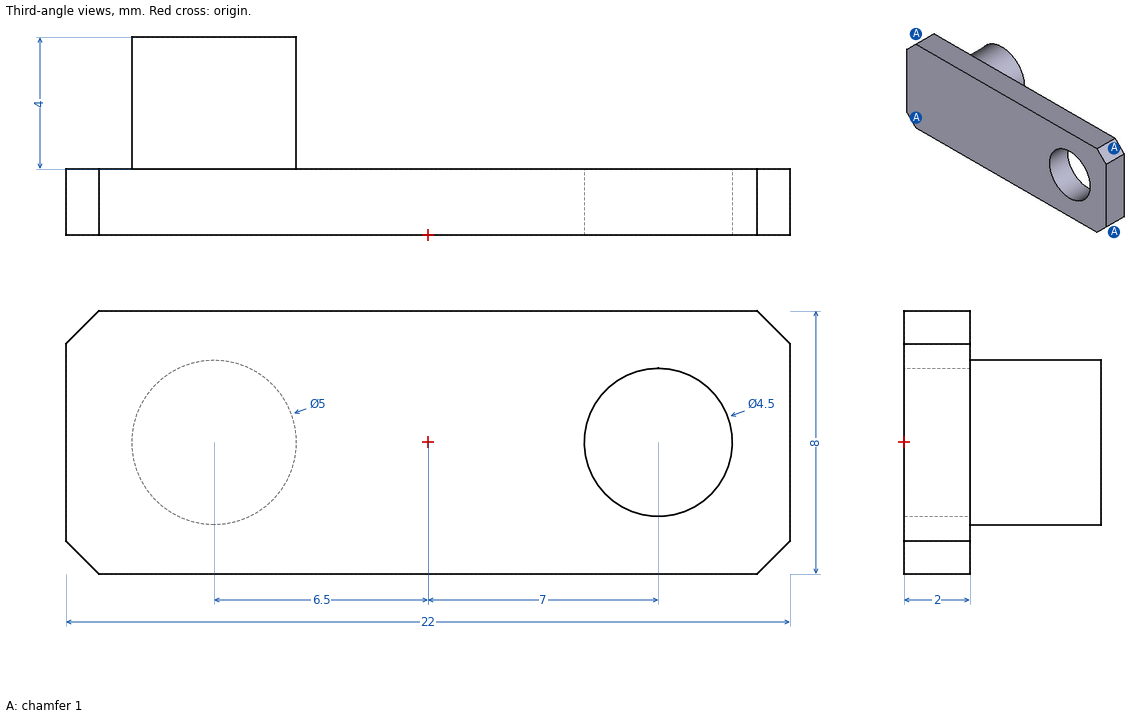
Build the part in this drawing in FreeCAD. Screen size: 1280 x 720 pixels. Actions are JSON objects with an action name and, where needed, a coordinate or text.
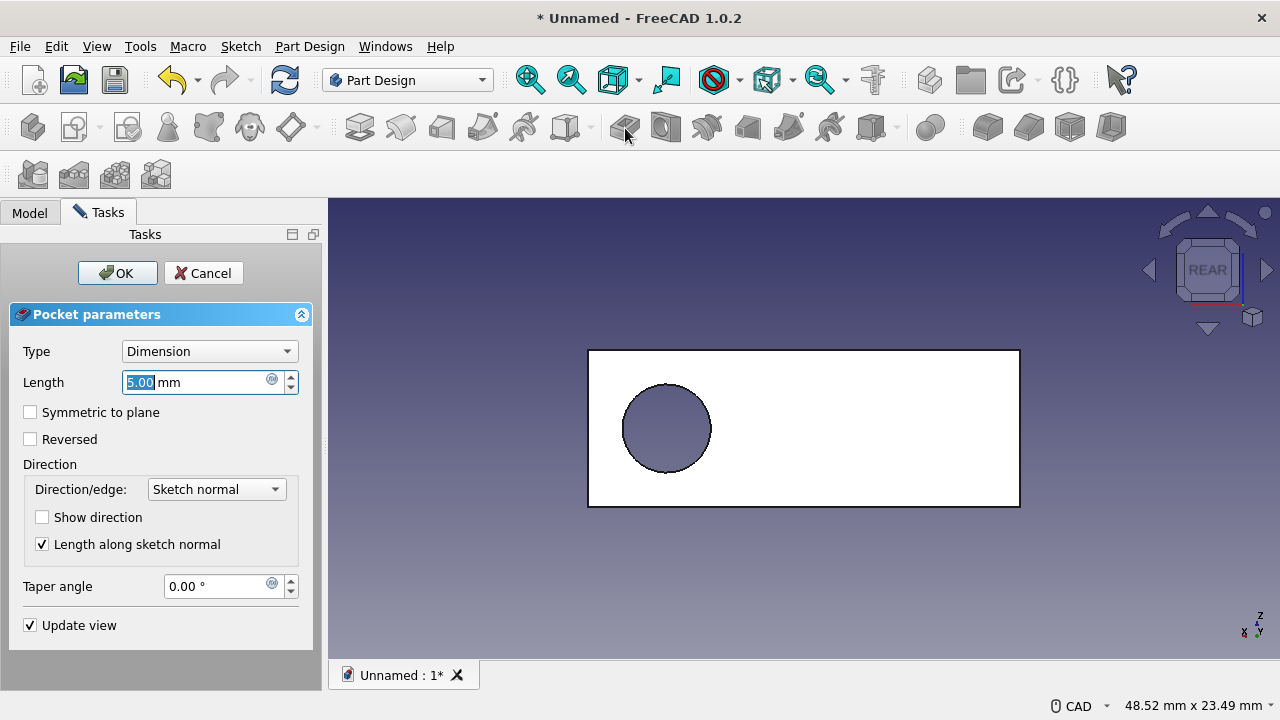
{"action": "left_click", "coordinate": [210, 352]}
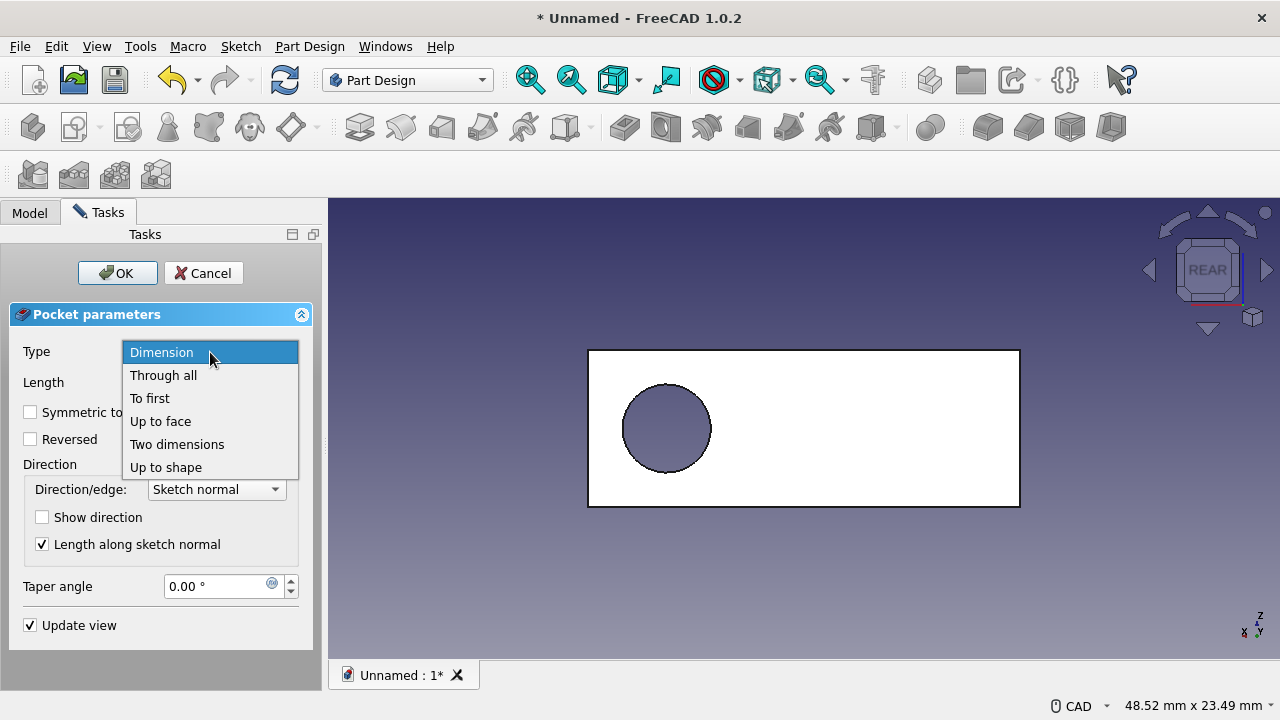
{"action": "left_click", "coordinate": [208, 376]}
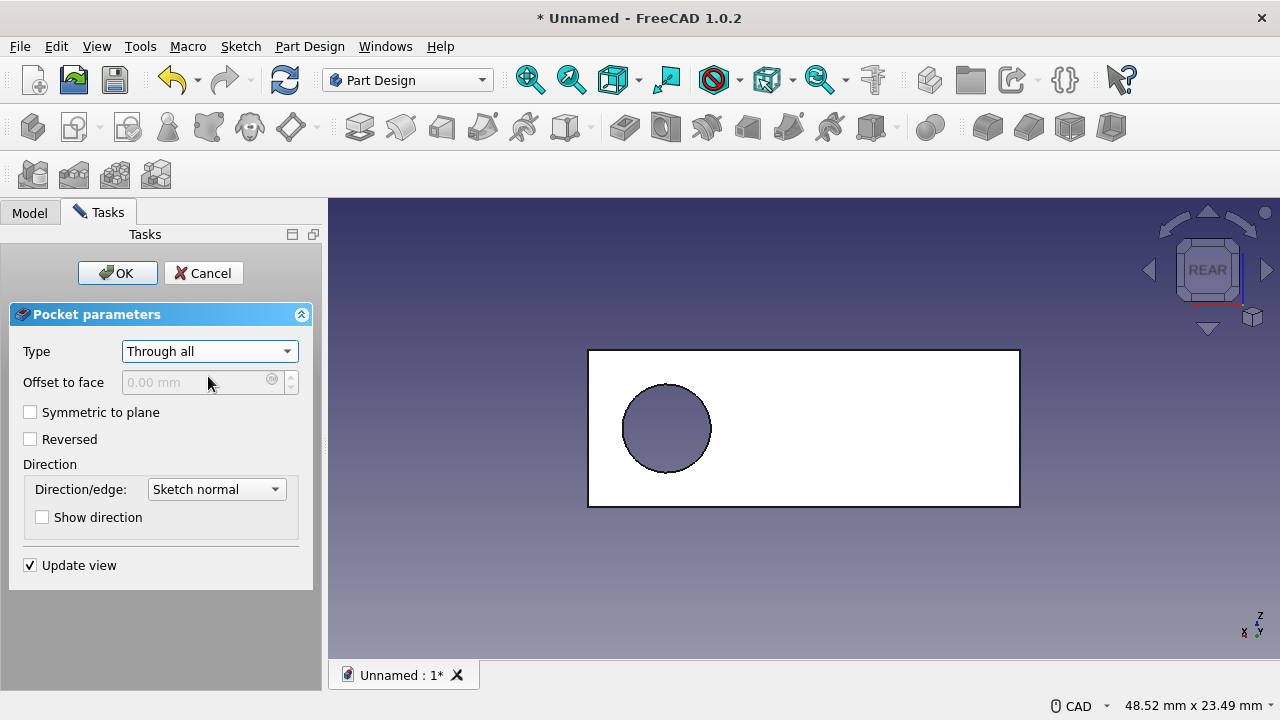
{"action": "left_click", "coordinate": [118, 273]}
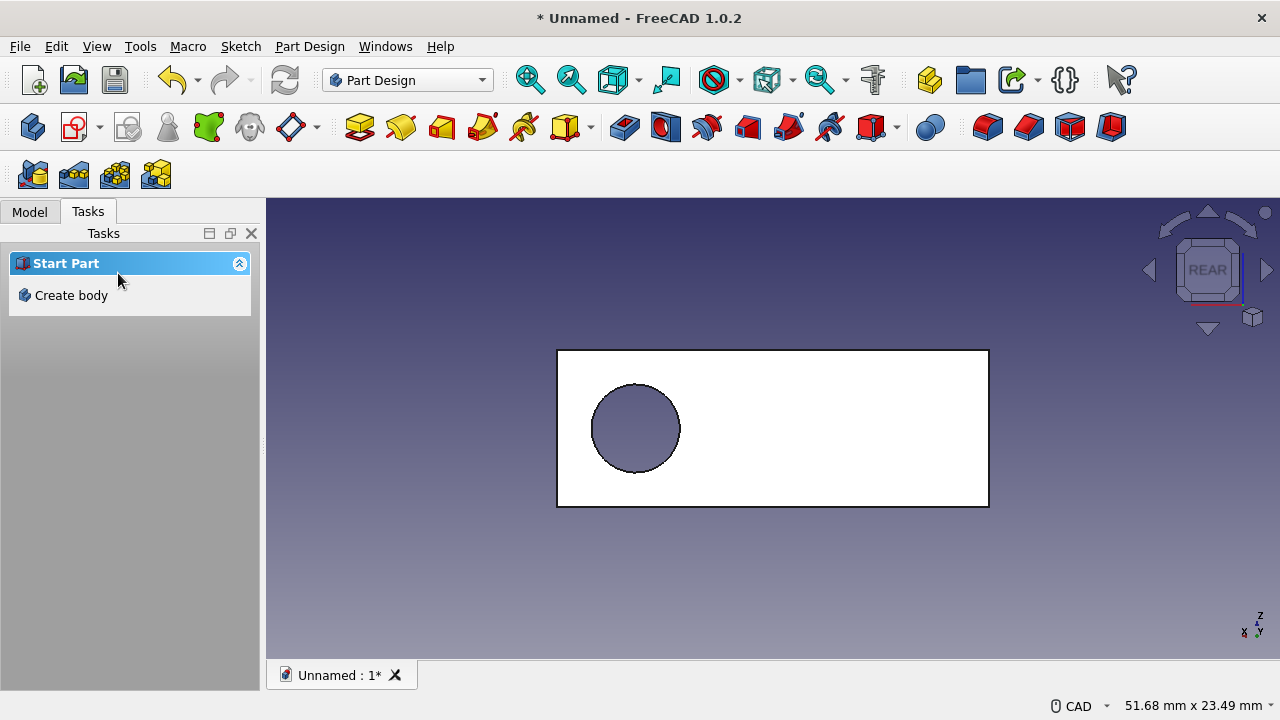
{"action": "key", "text": "v f"}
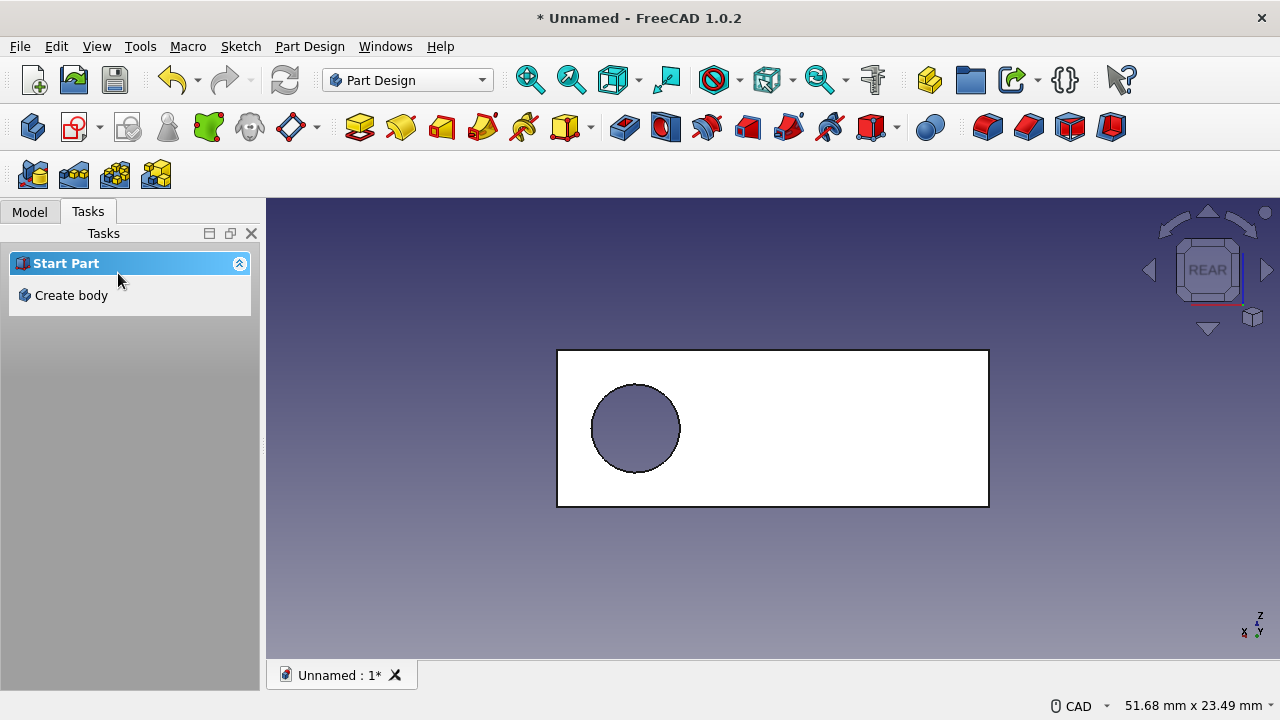
{"action": "left_click", "coordinate": [773, 427]}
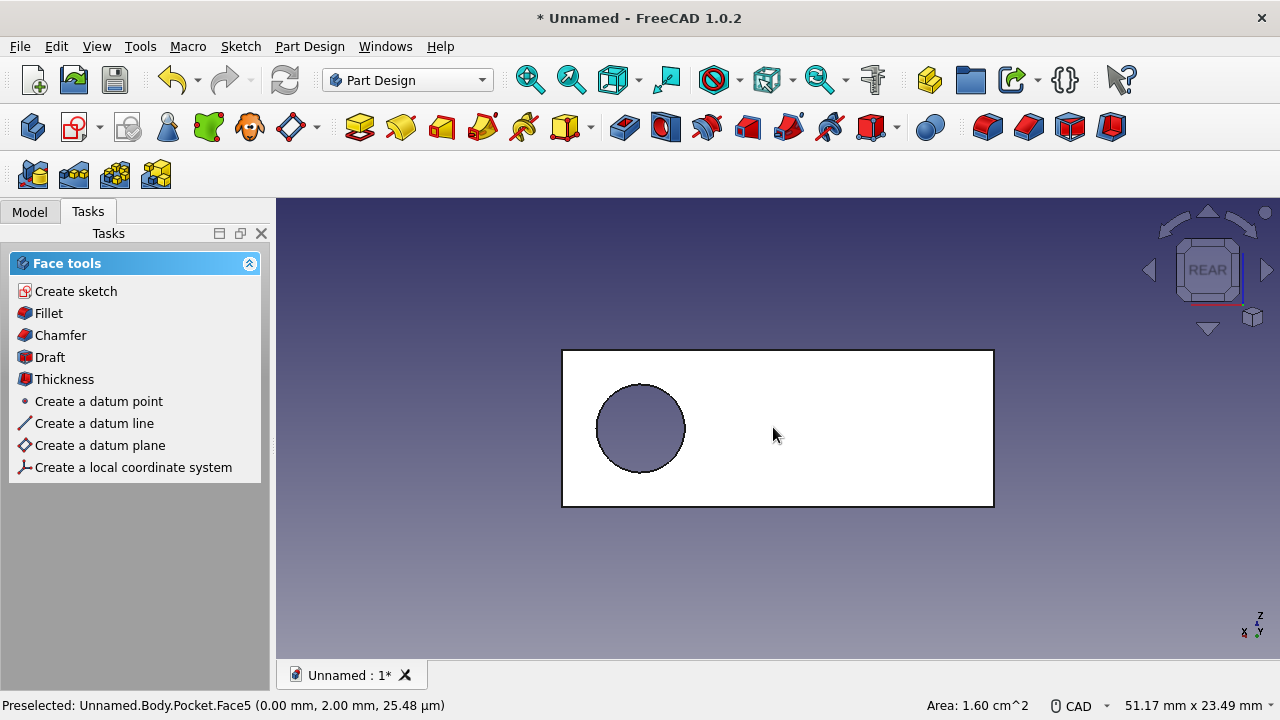
{"action": "left_click", "coordinate": [74, 128]}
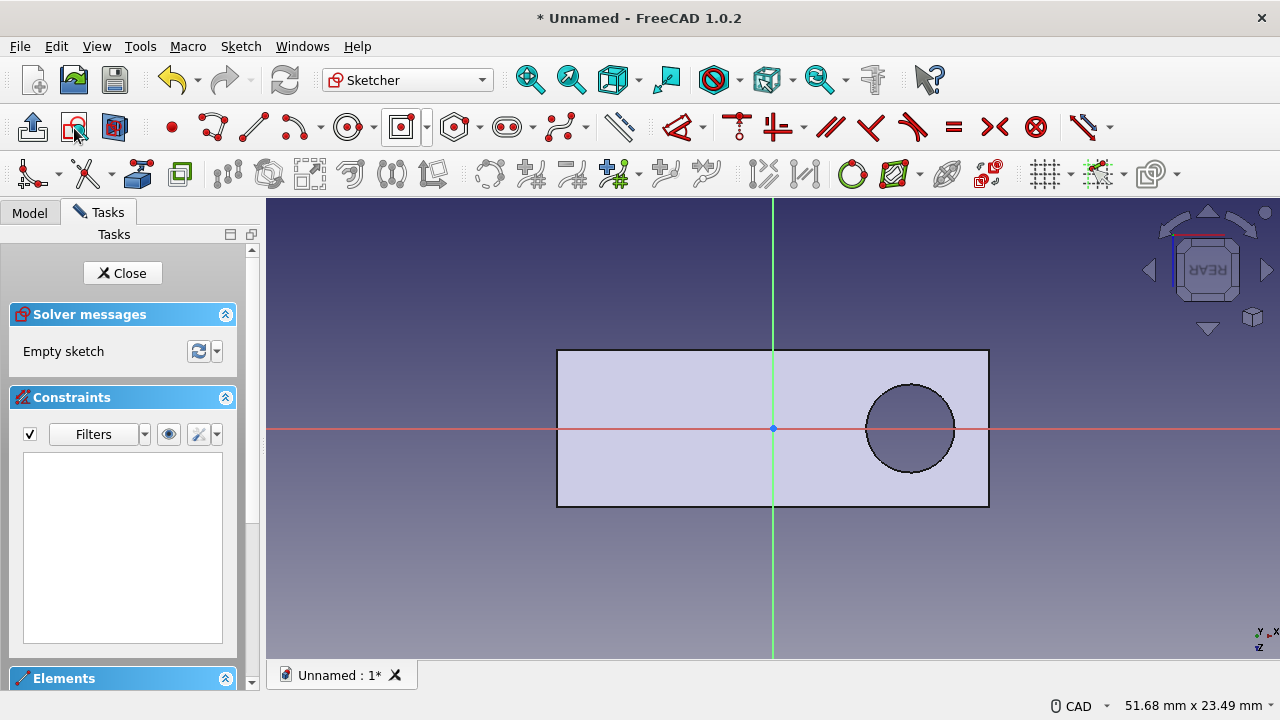
{"action": "scroll", "coordinate": [673, 428], "scroll_direction": "up", "scroll_amount": 5}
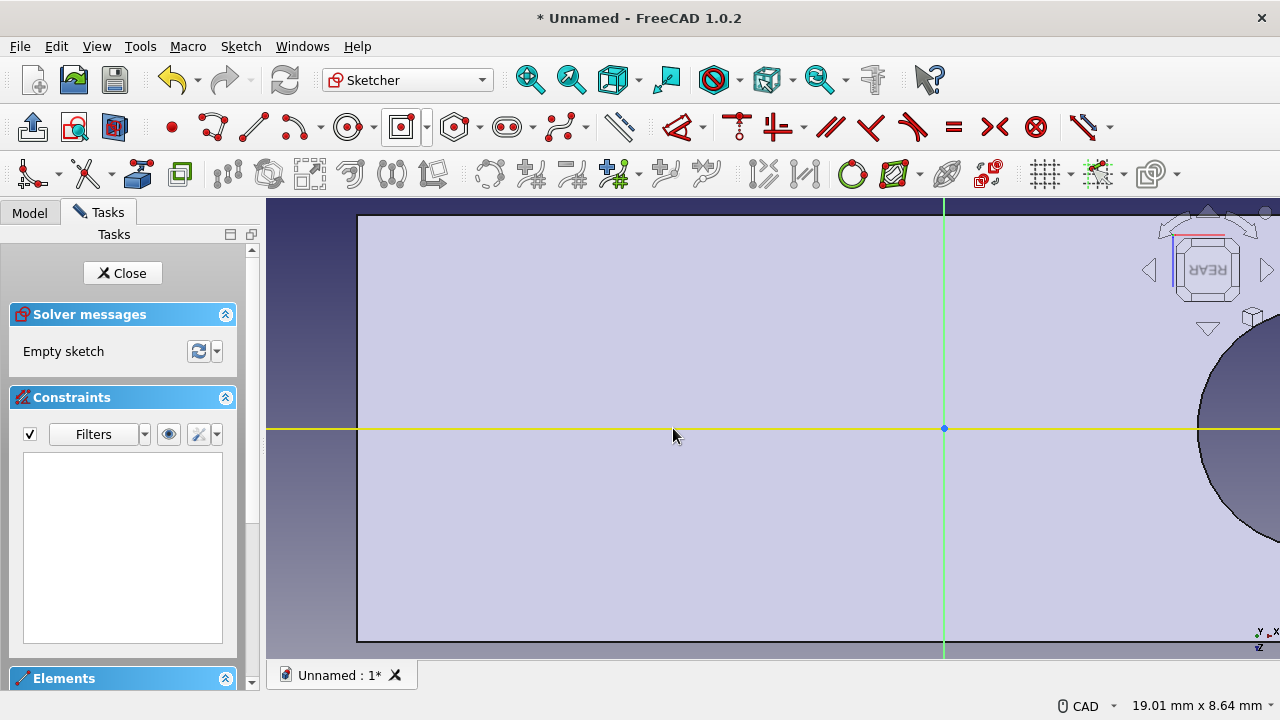
{"action": "left_click", "coordinate": [348, 128]}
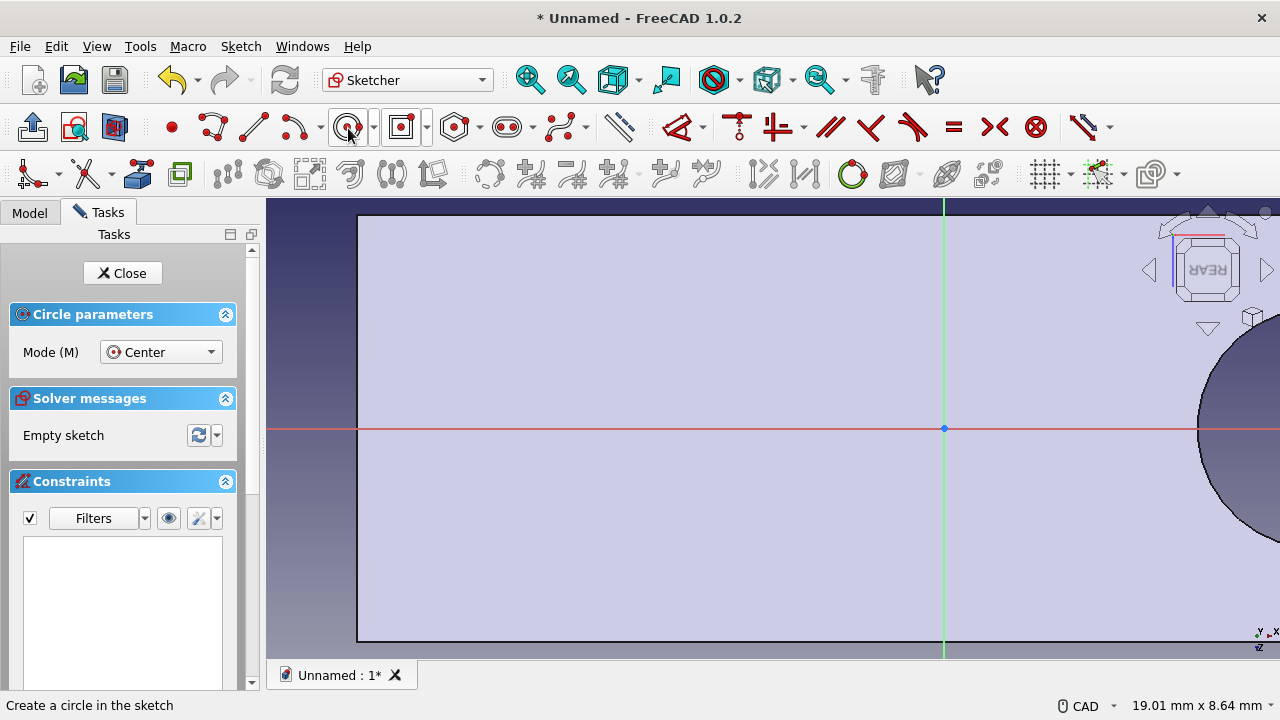
{"action": "left_click", "coordinate": [597, 428]}
{"action": "left_click", "coordinate": [692, 334]}
{"action": "key", "text": "Escape"}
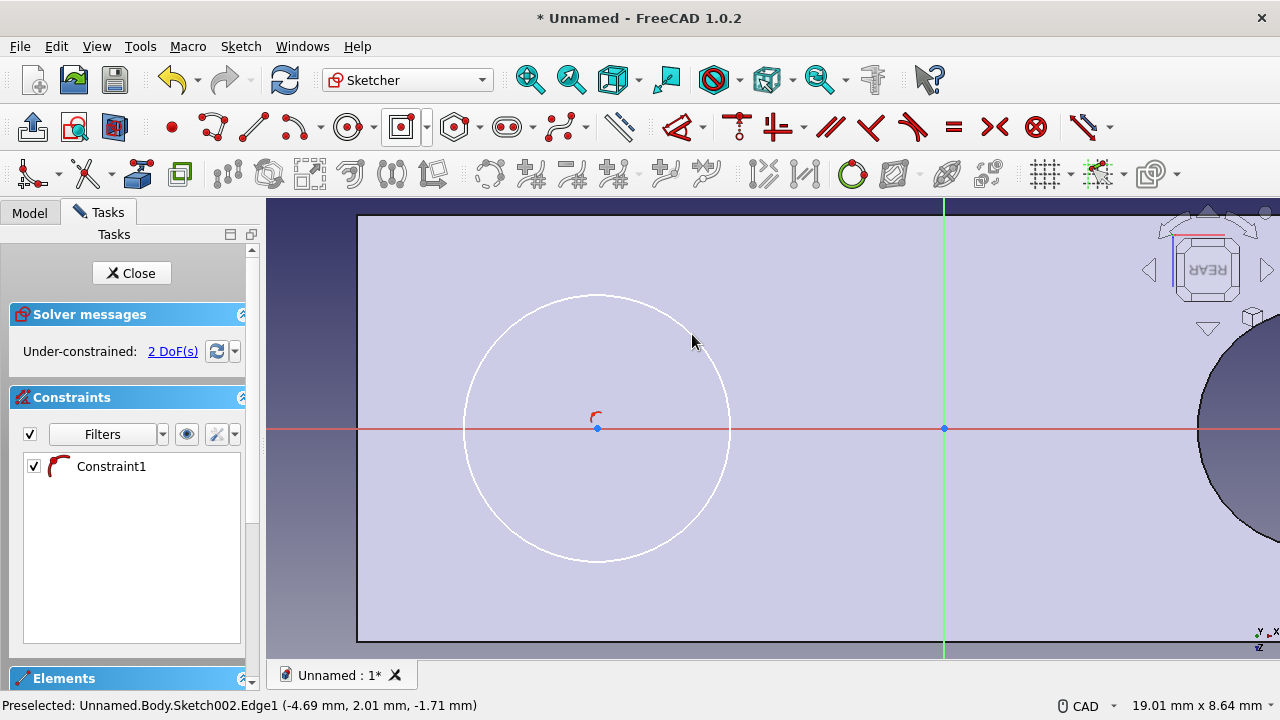
{"action": "left_click", "coordinate": [676, 128]}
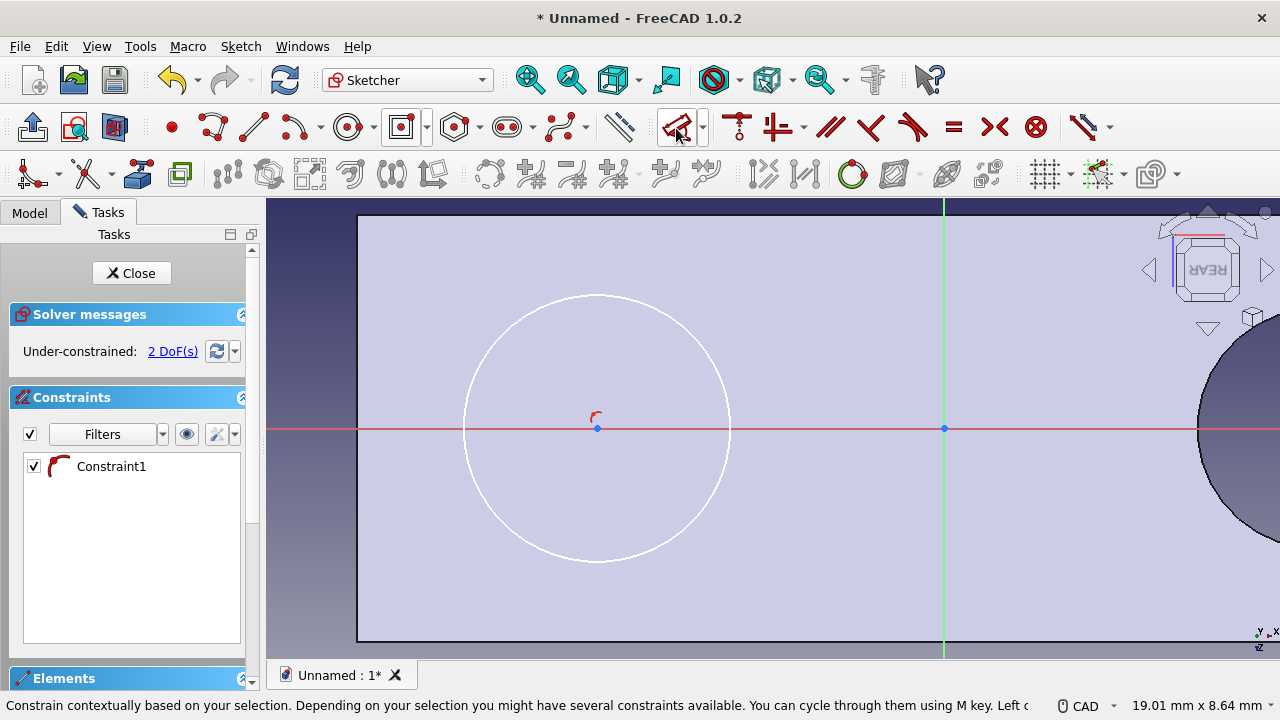
{"action": "left_click", "coordinate": [691, 334]}
{"action": "left_click", "coordinate": [714, 311]}